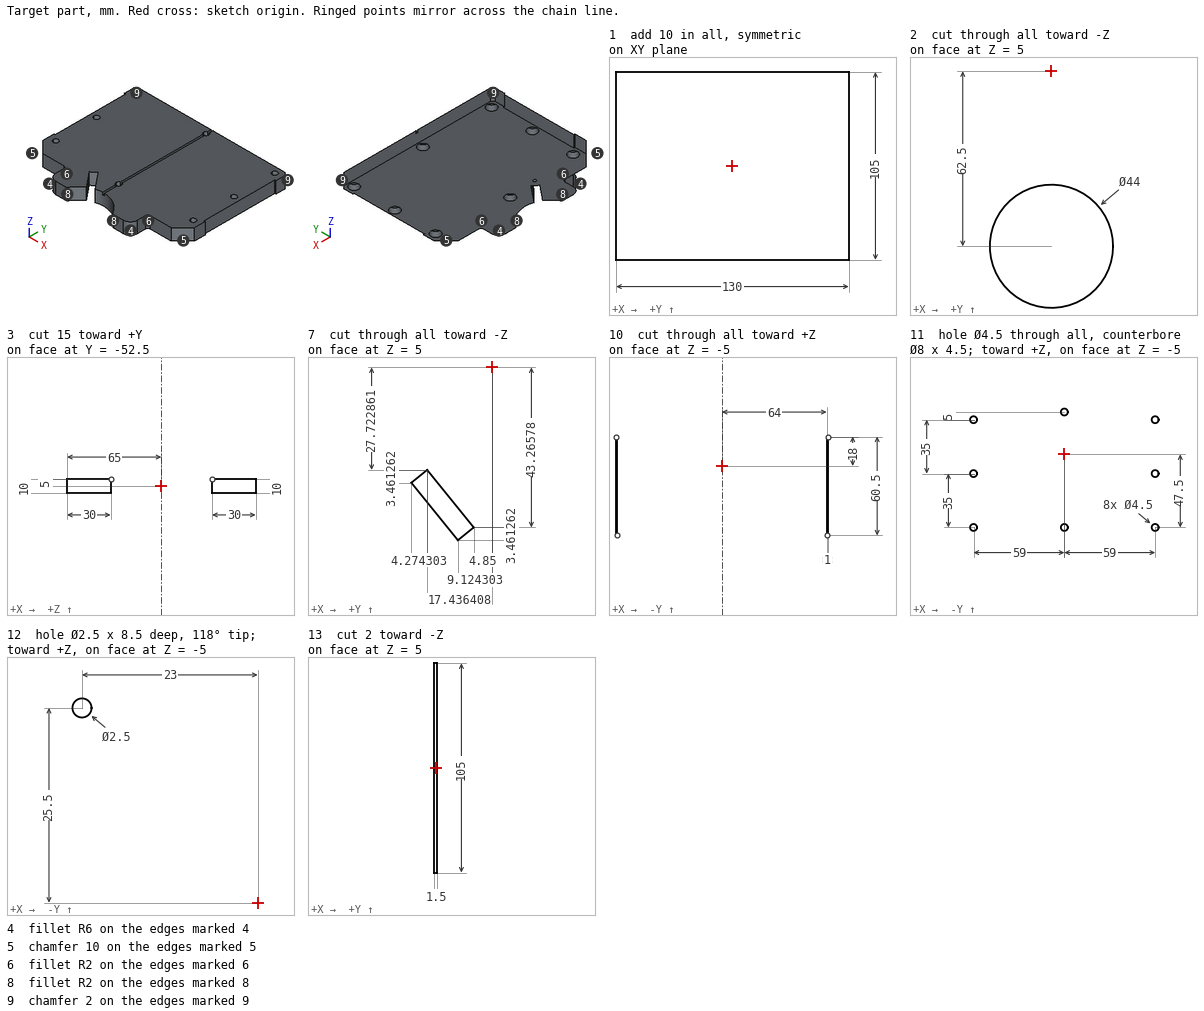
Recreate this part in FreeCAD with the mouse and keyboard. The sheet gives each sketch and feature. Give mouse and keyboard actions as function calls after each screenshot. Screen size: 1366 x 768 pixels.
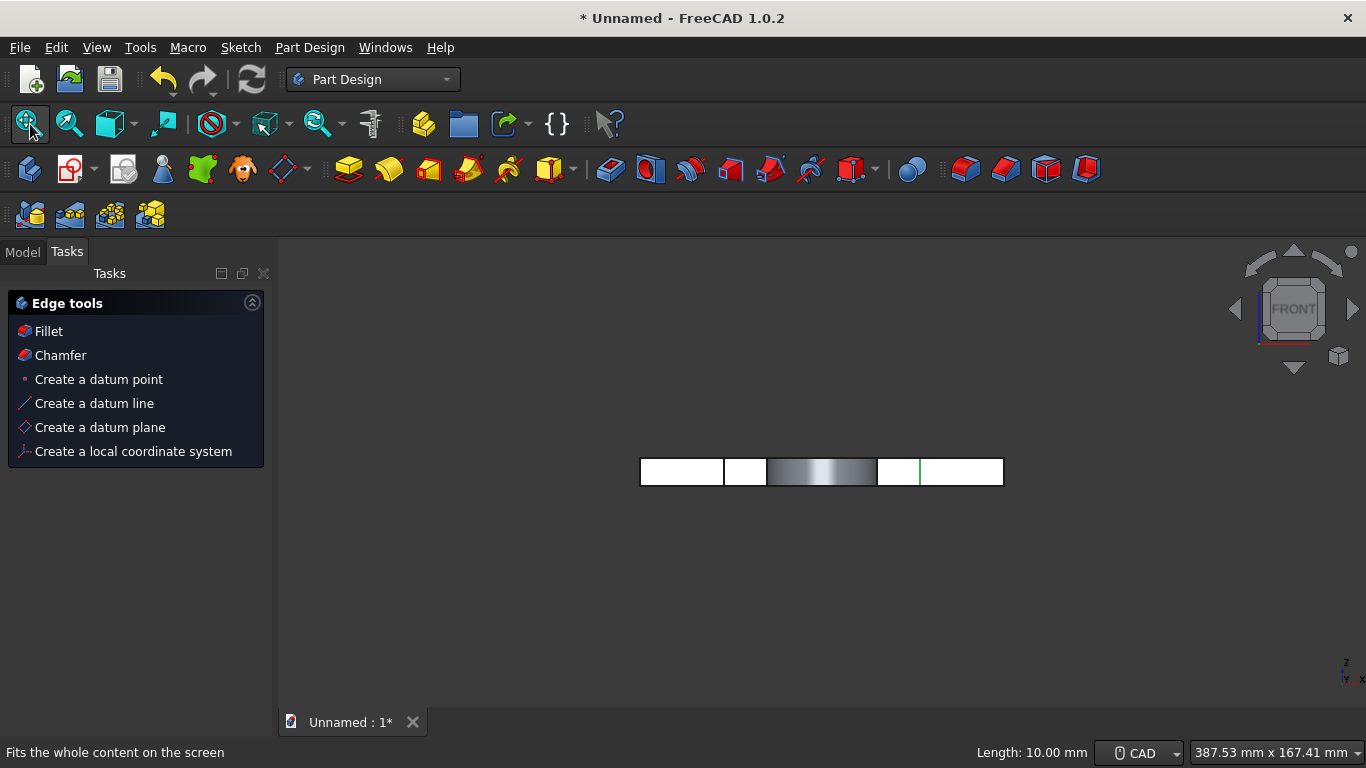
click(724, 471, ctrl)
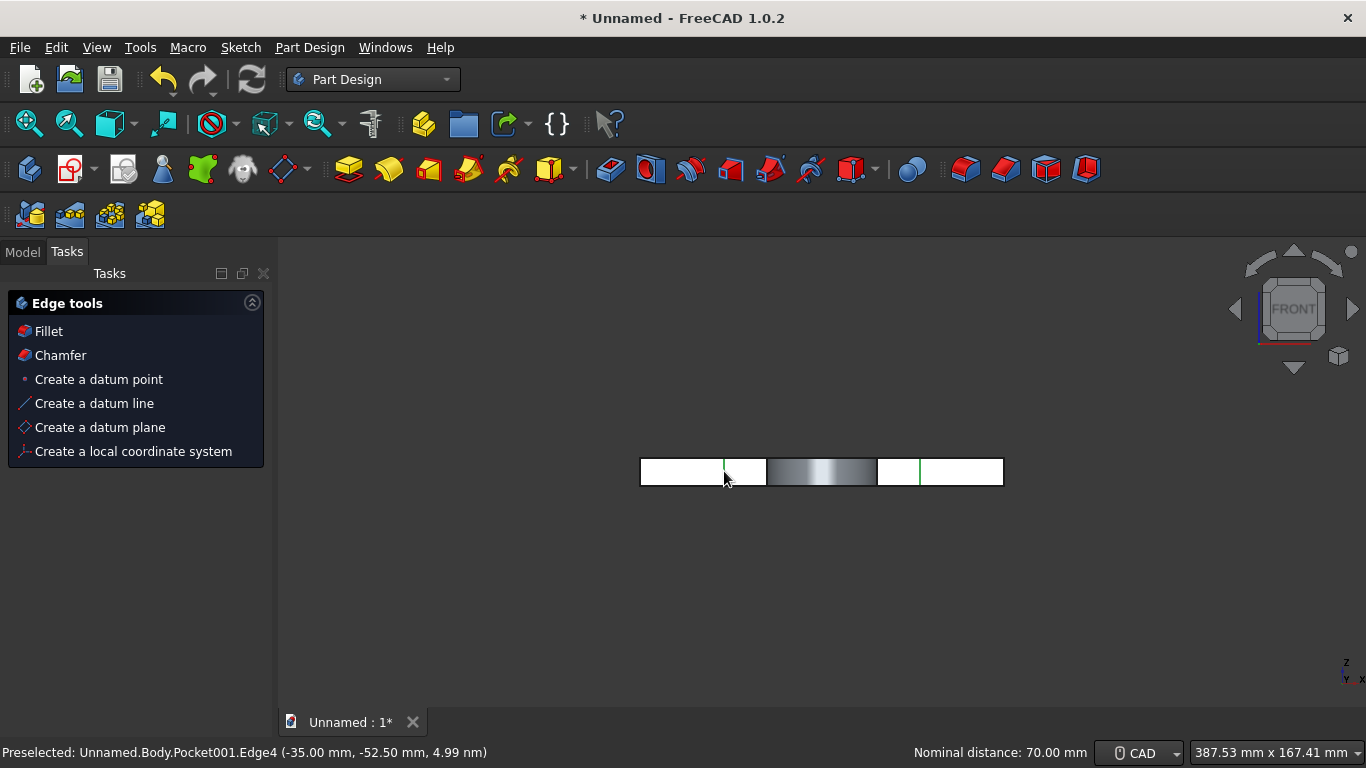
click(966, 170)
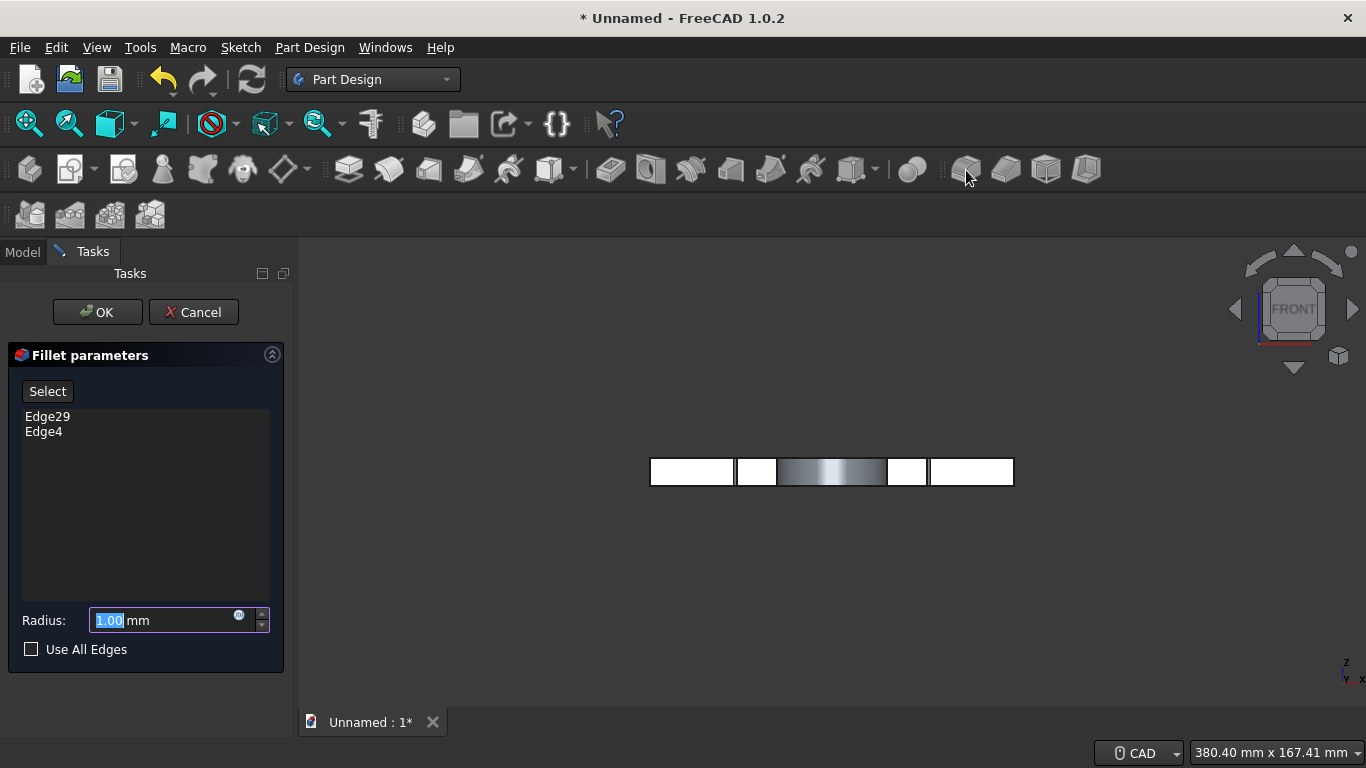
text(6)
key(Tab)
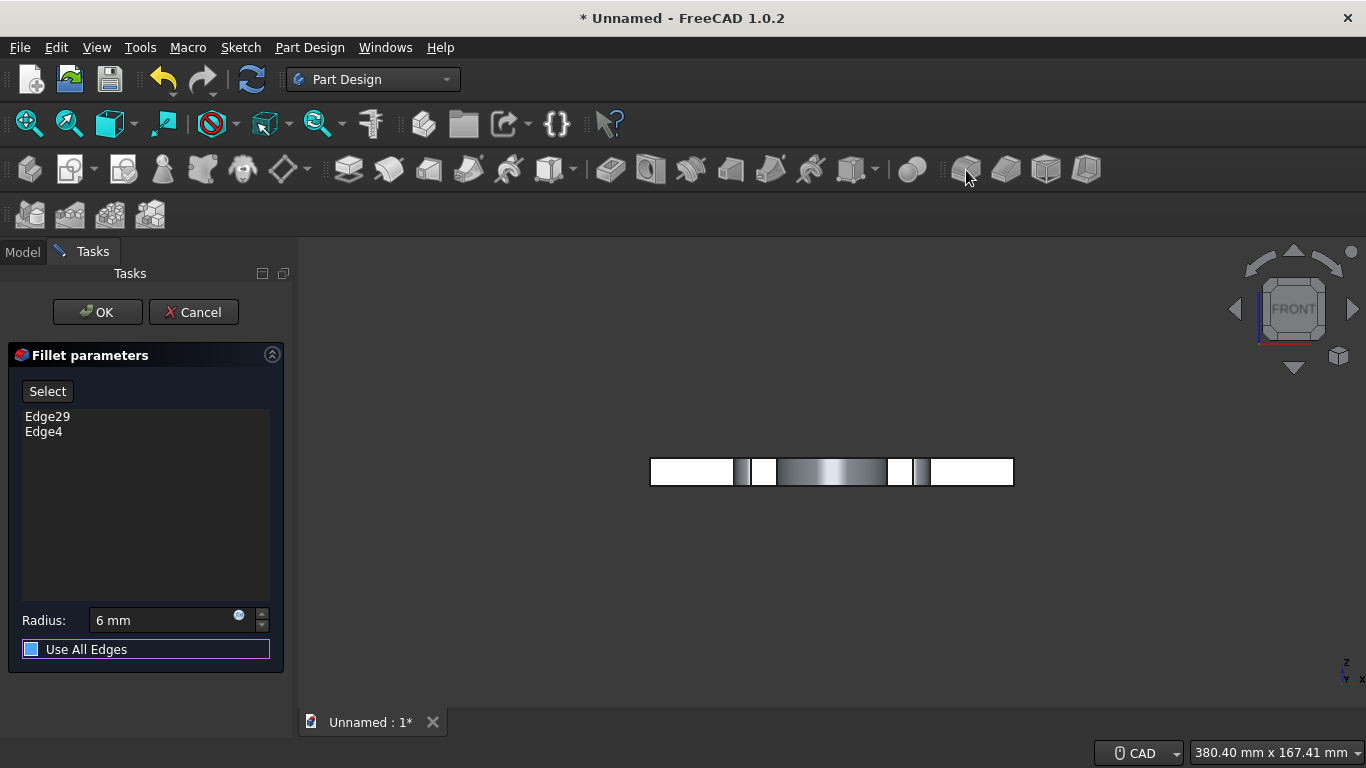
click(98, 312)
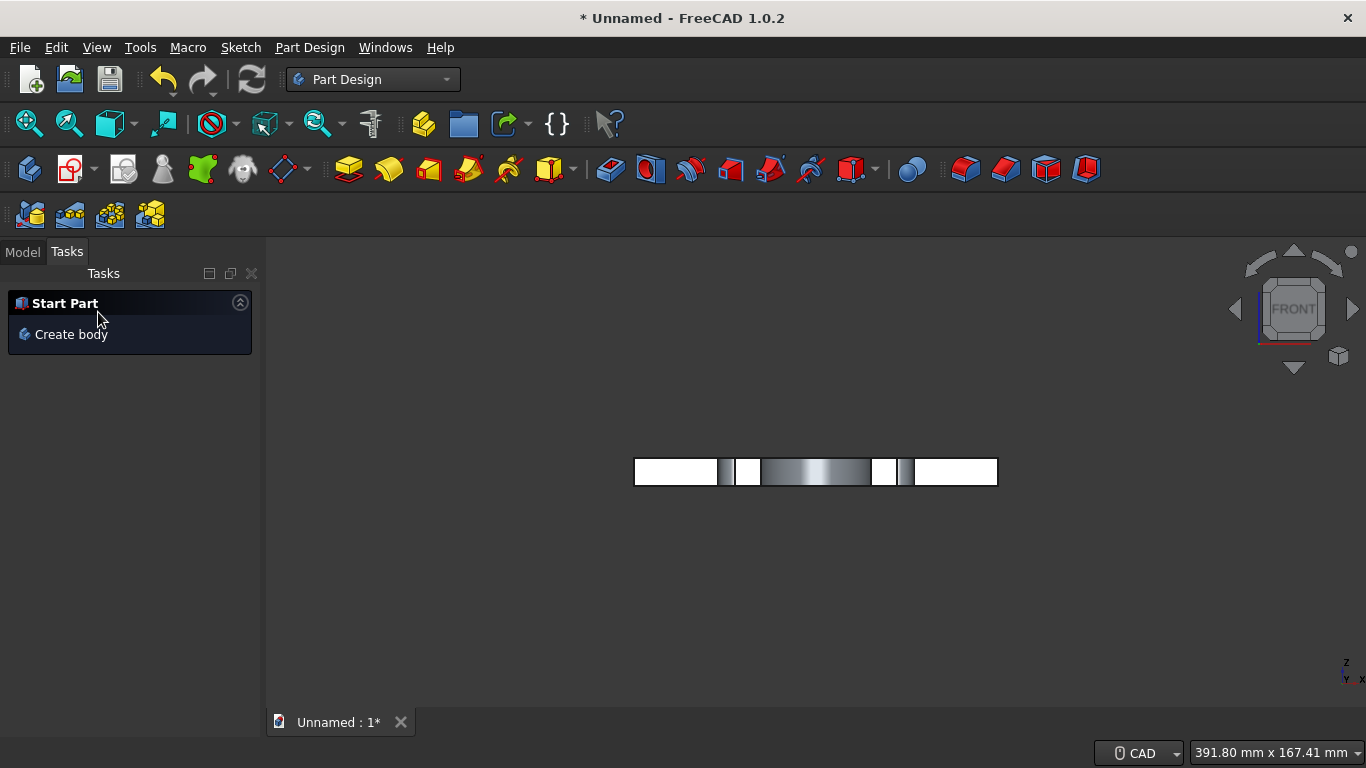
click(30, 124)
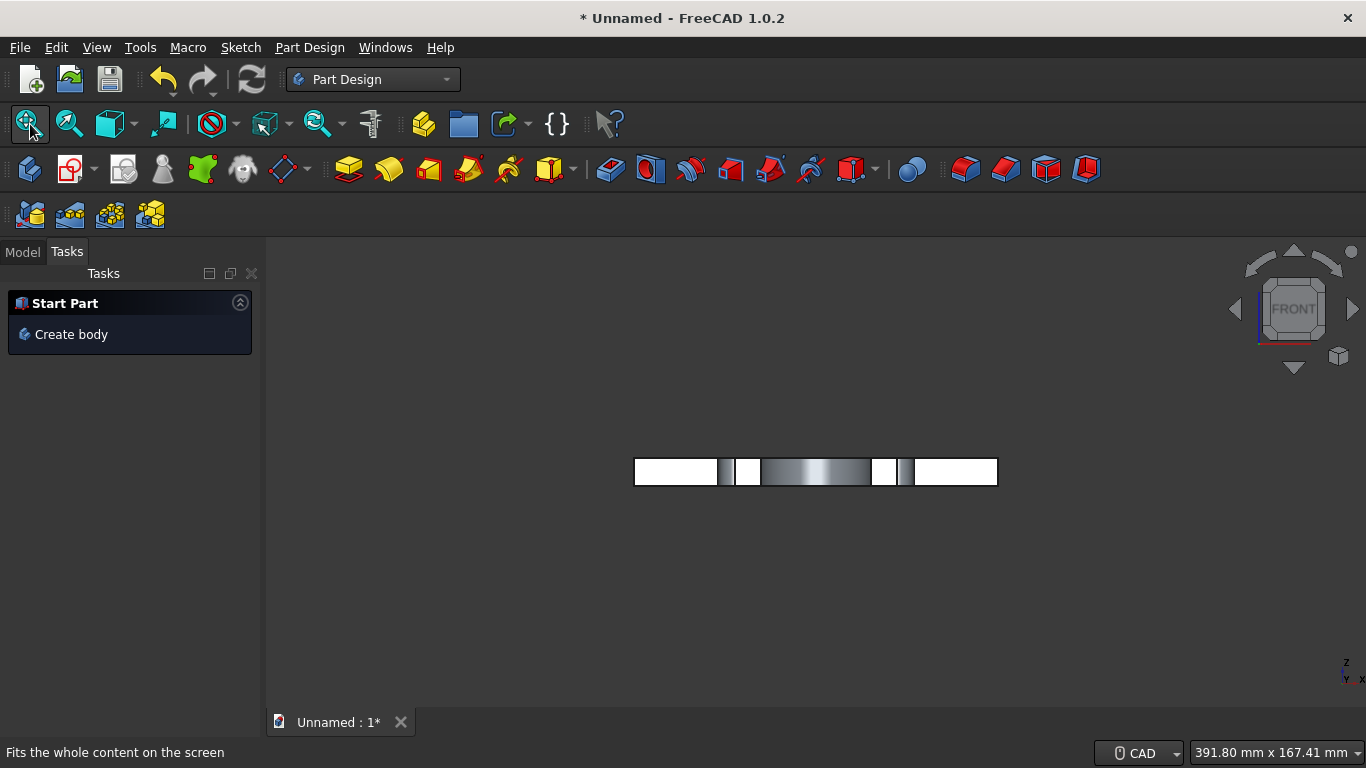
click(634, 471)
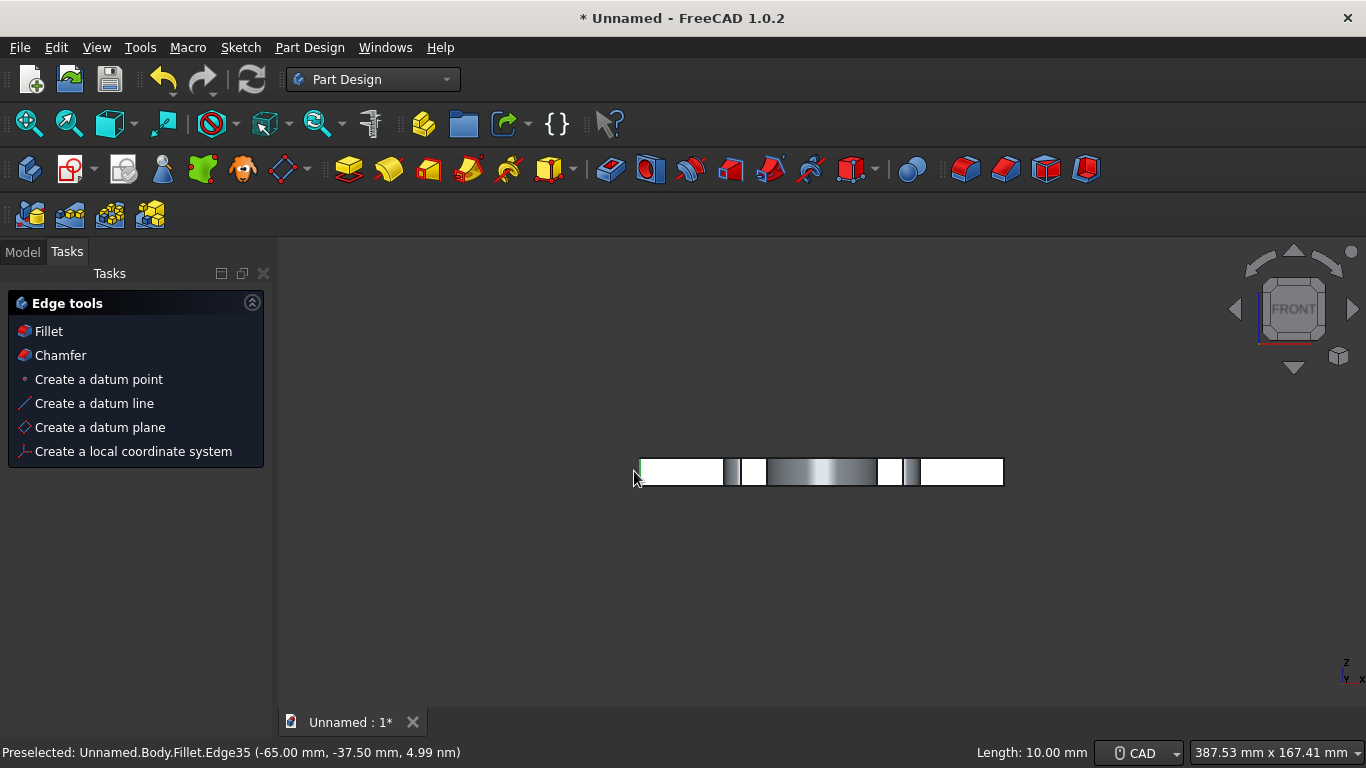
click(1004, 471, ctrl)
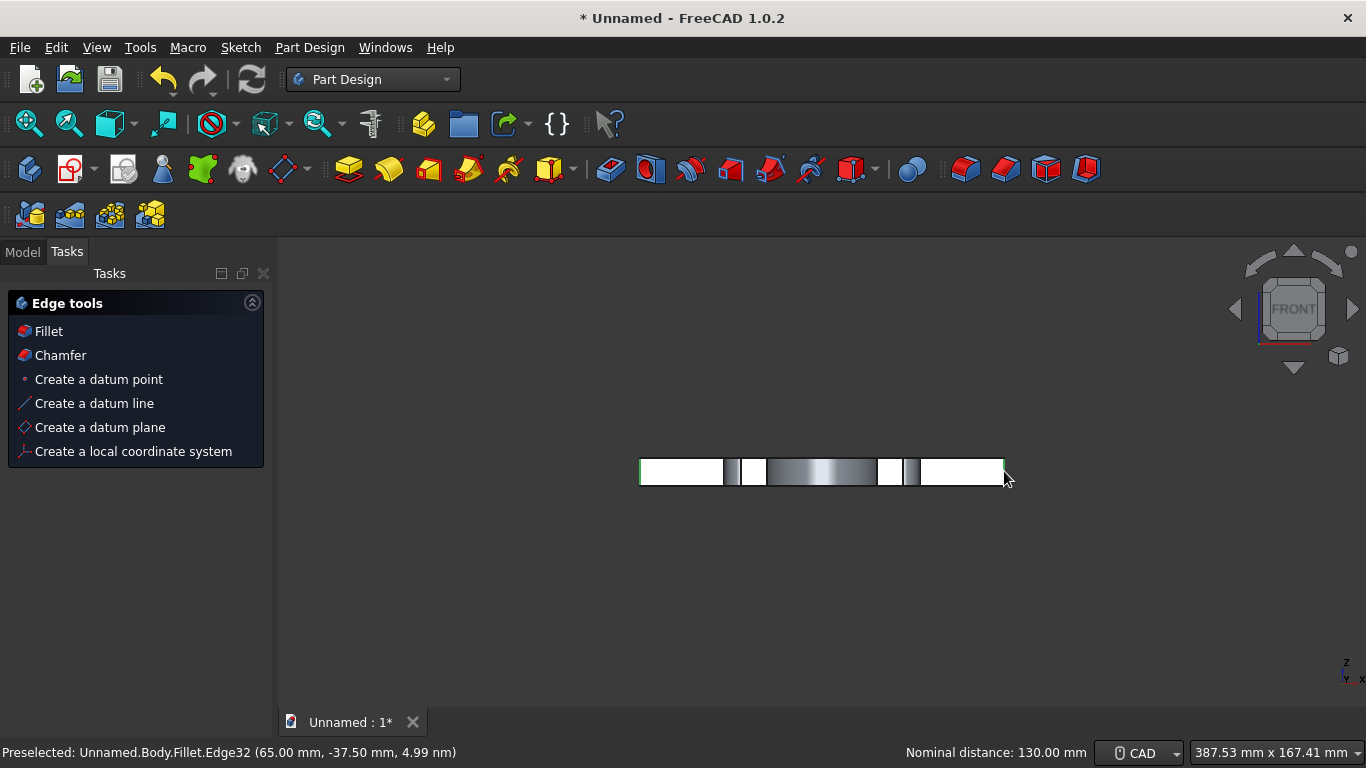
click(1006, 170)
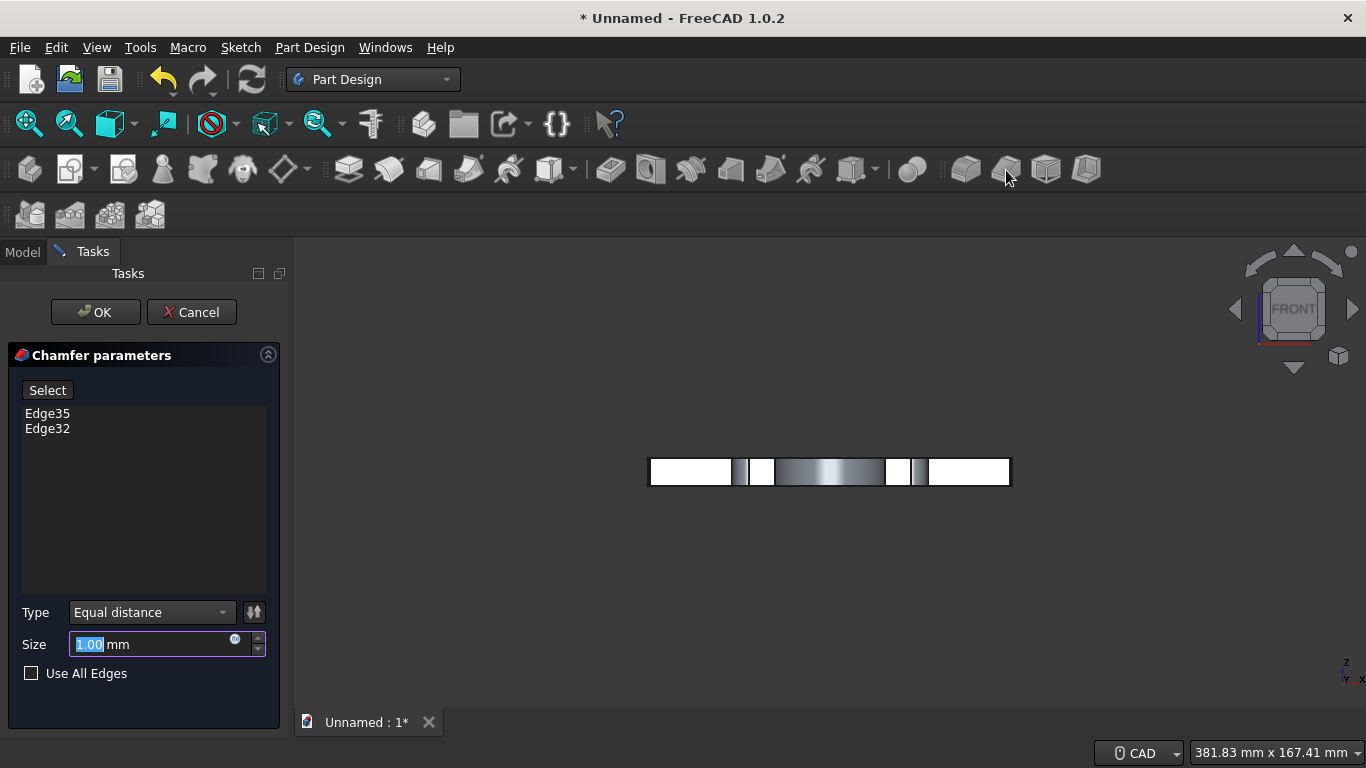
text(10)
key(Tab)